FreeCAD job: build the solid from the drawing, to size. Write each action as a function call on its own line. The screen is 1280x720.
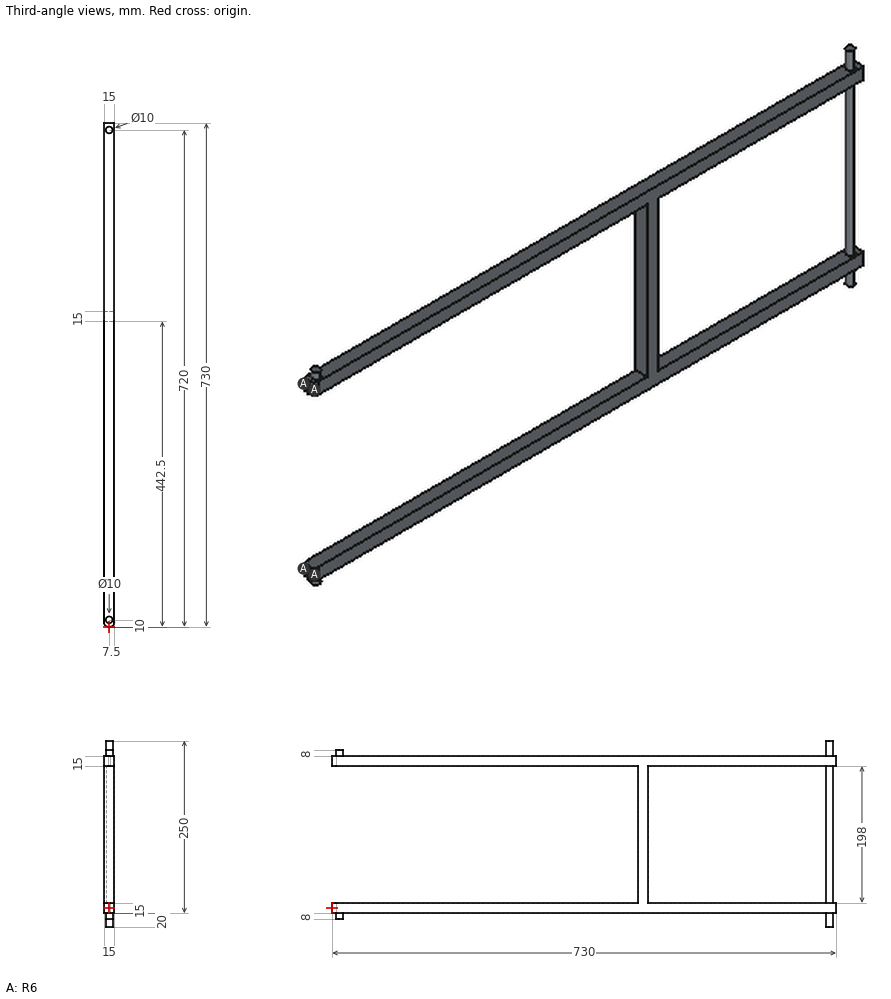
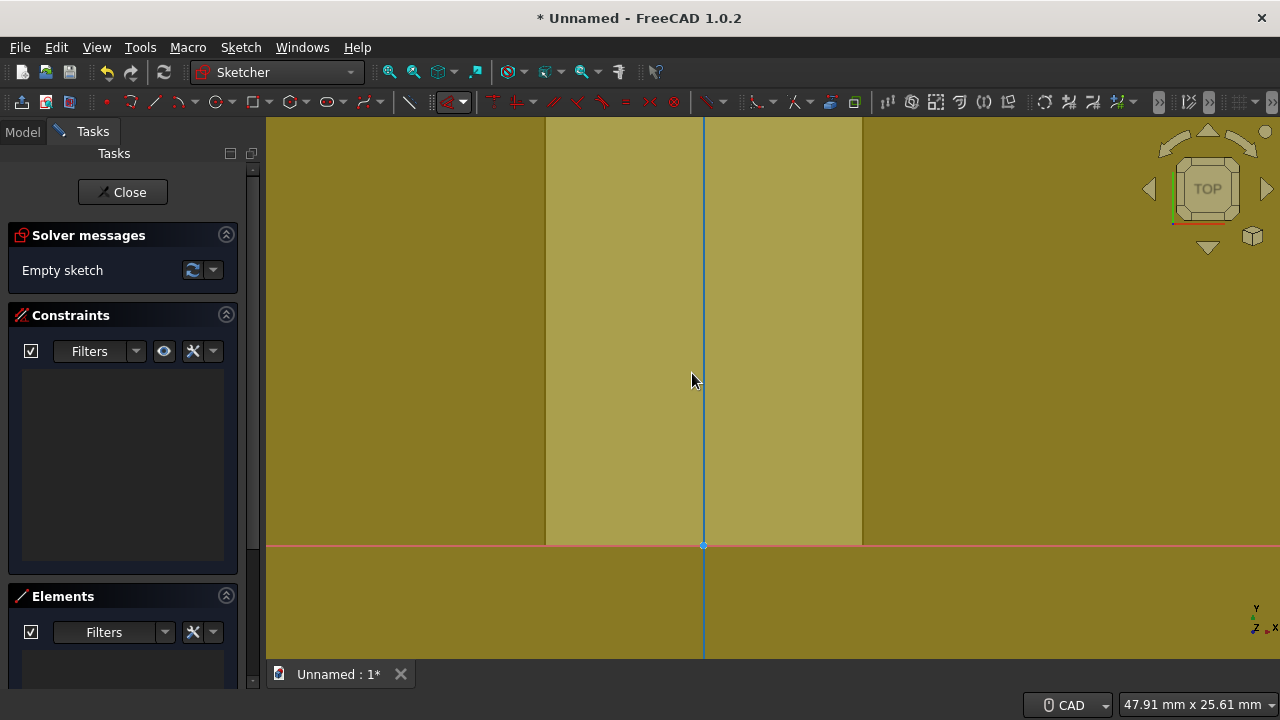
click(216, 102)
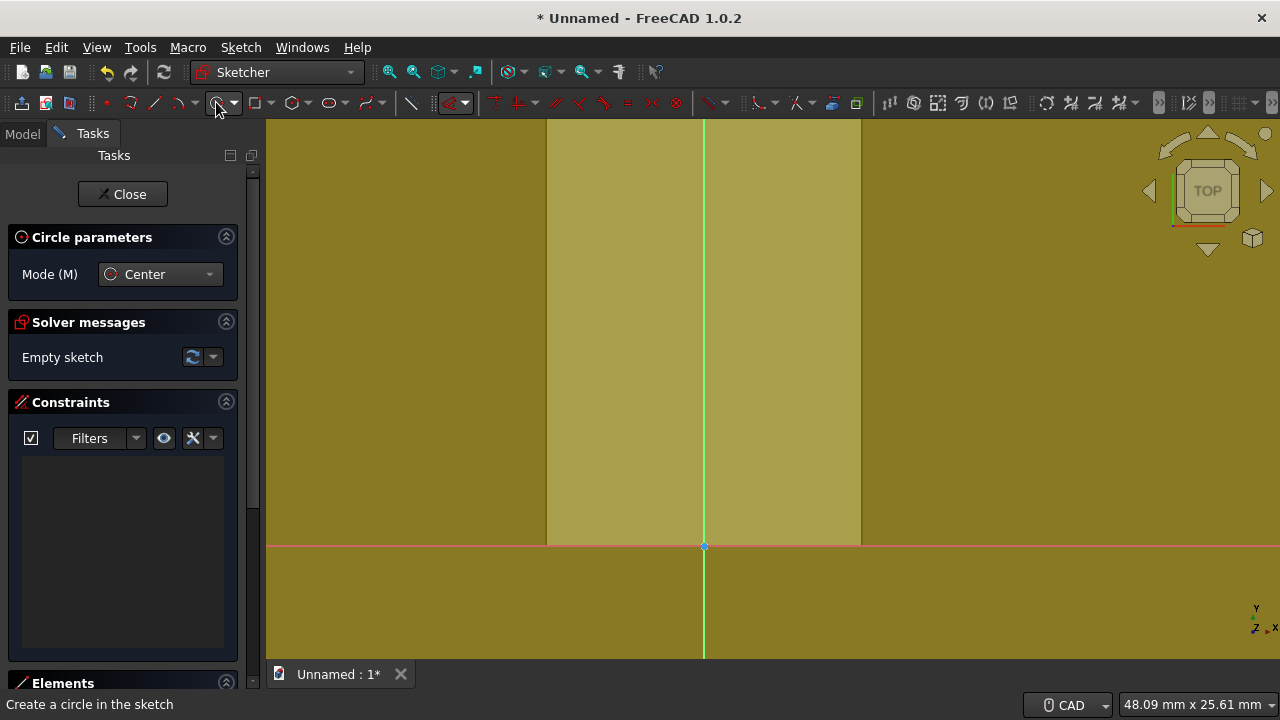
click(704, 335)
move(779, 261)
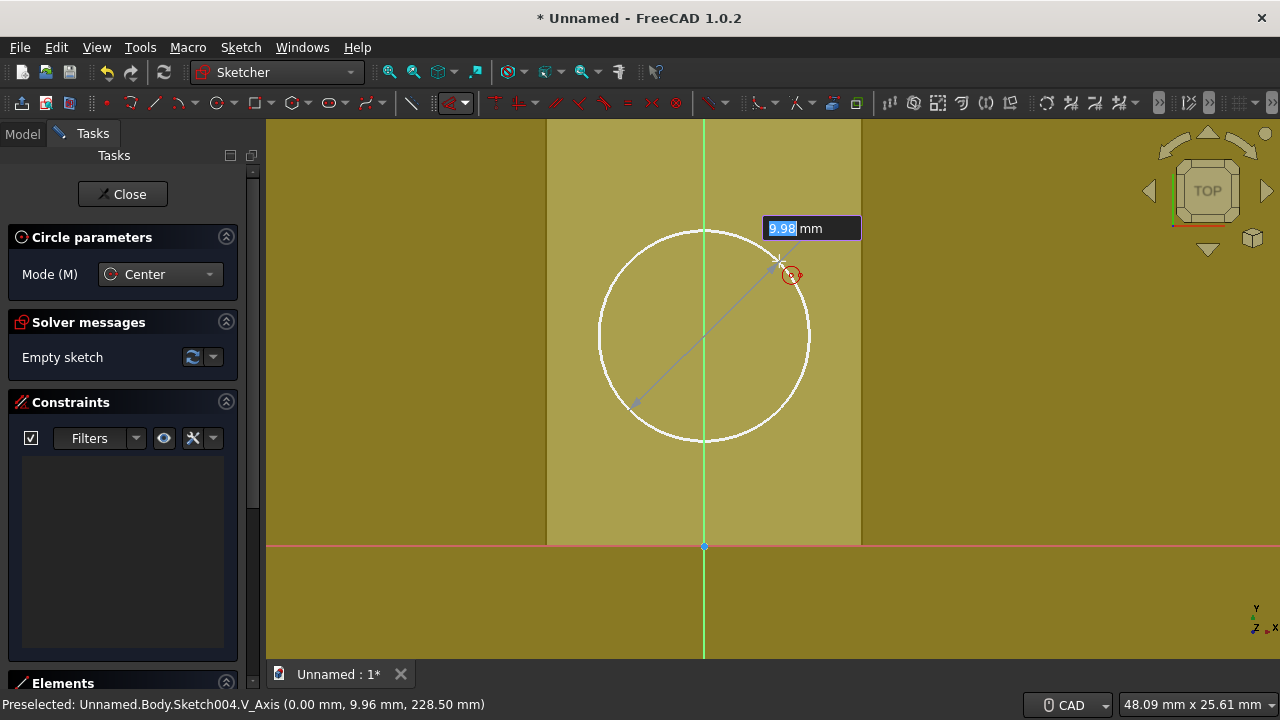
text(10)
key(Return)
key(Escape)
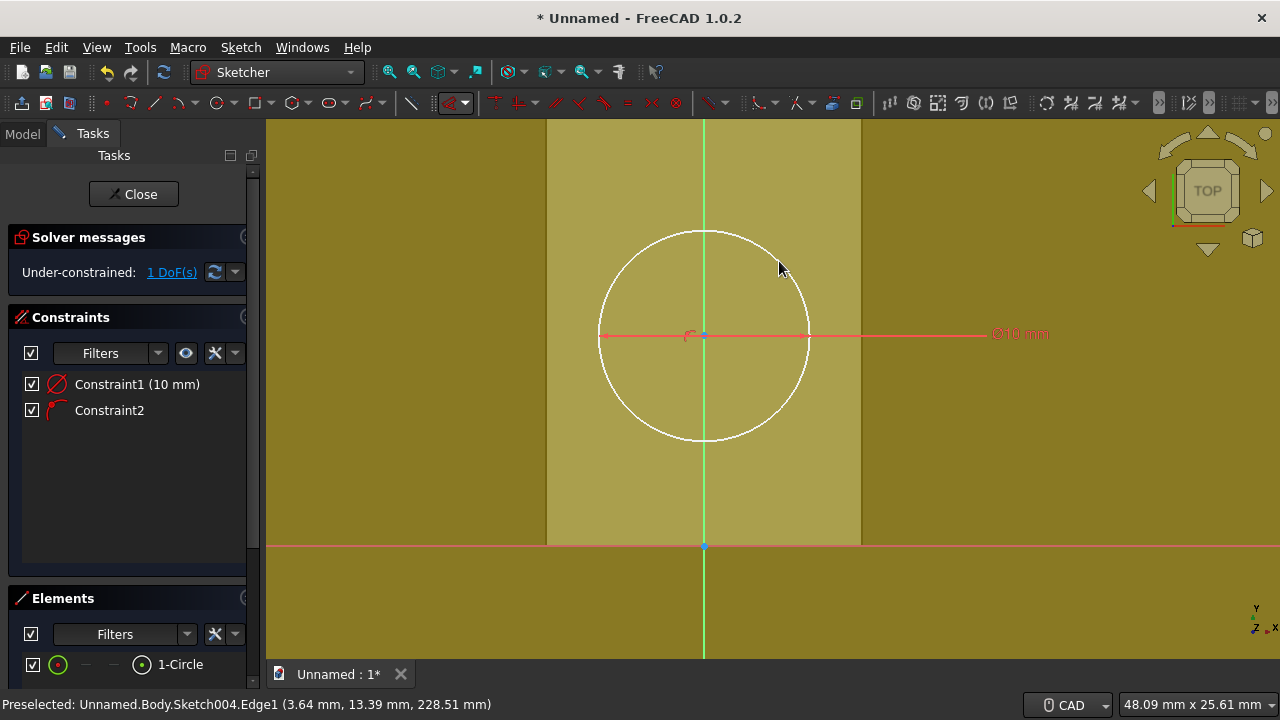
click(704, 336)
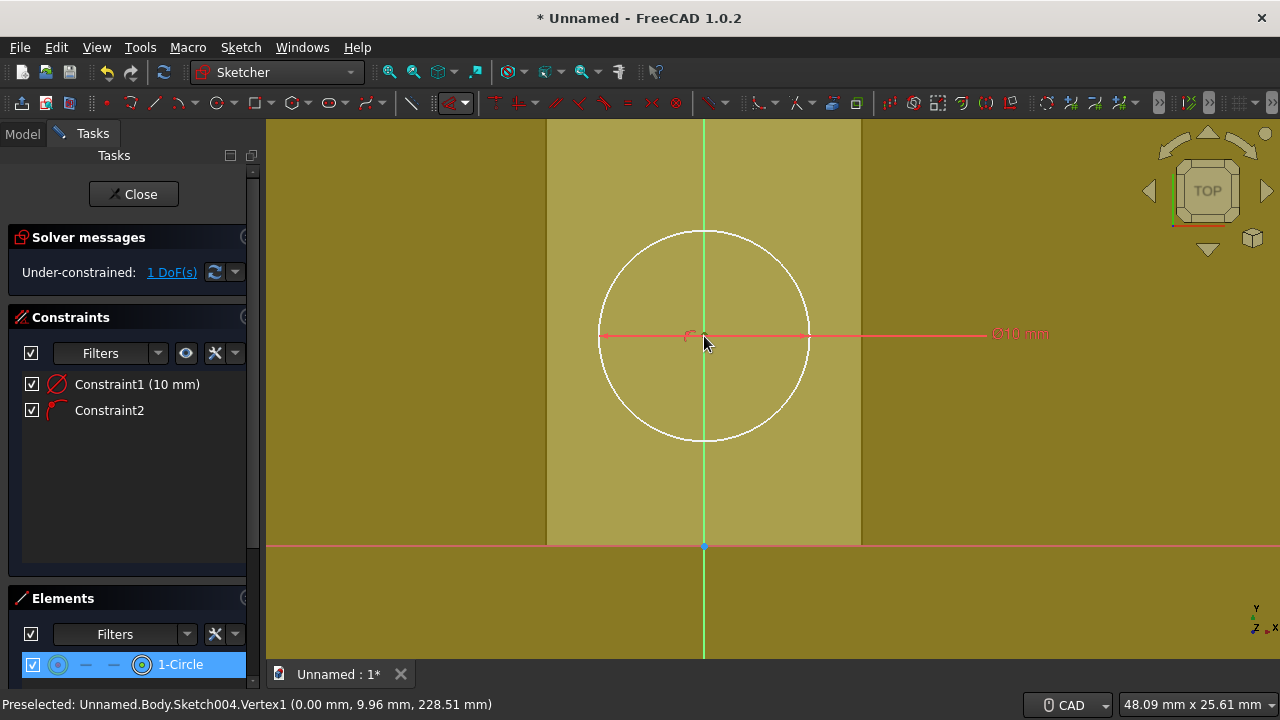
key(i)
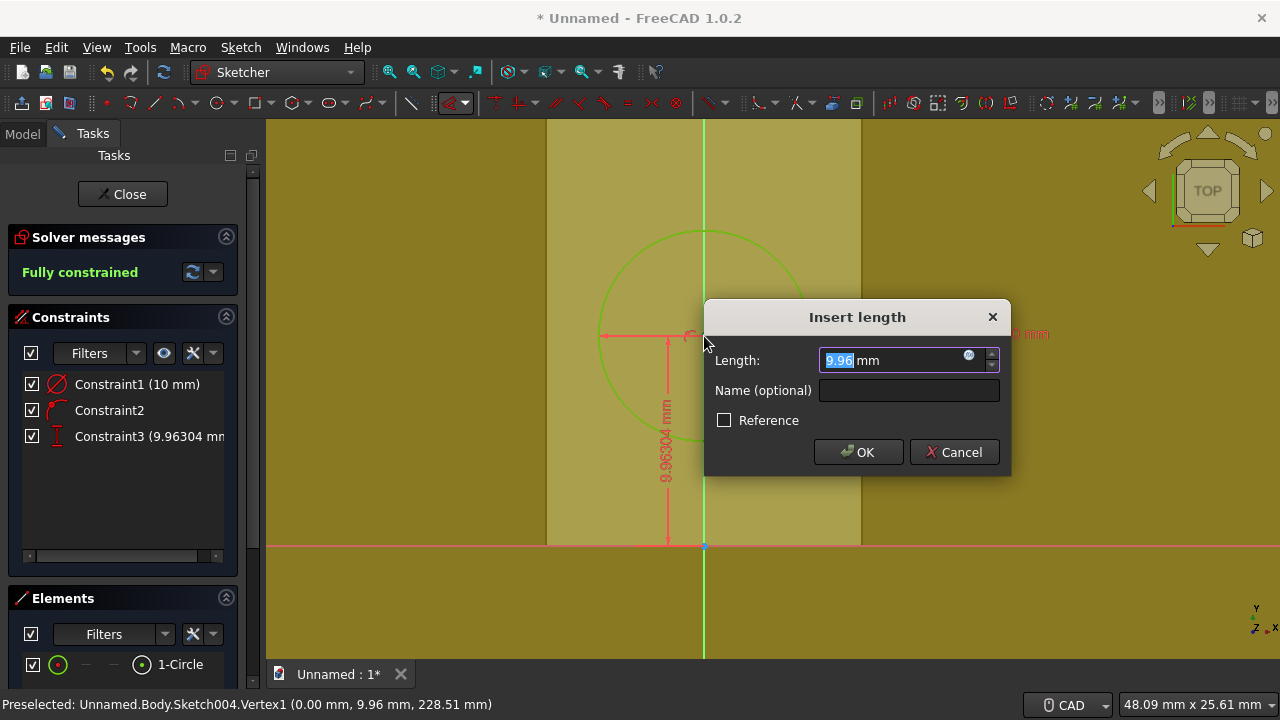
text(10)
key(Return)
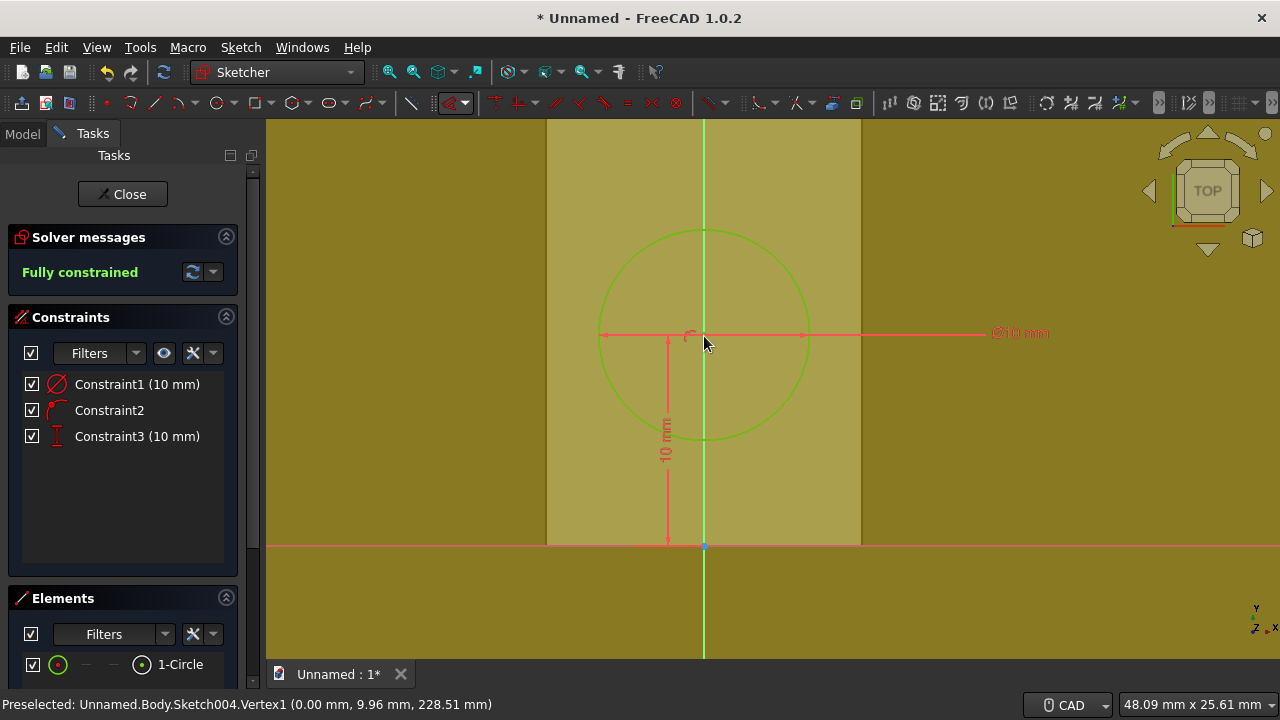
click(123, 194)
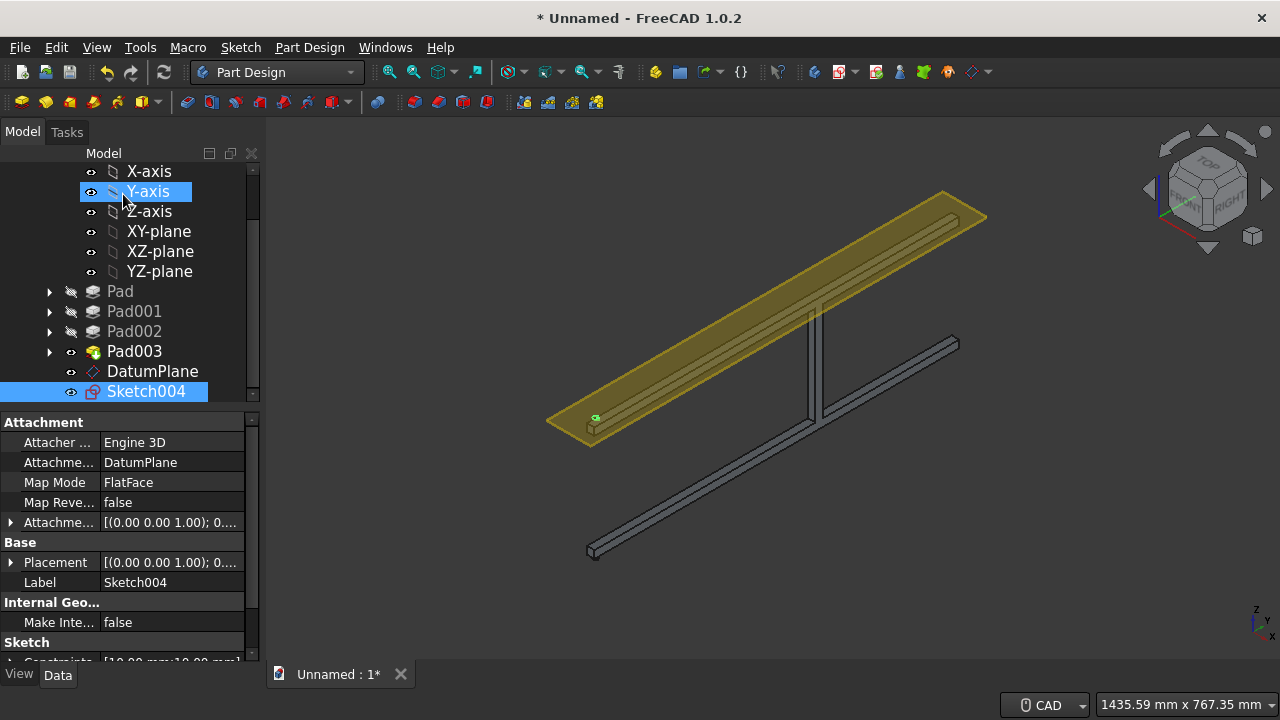
click(22, 102)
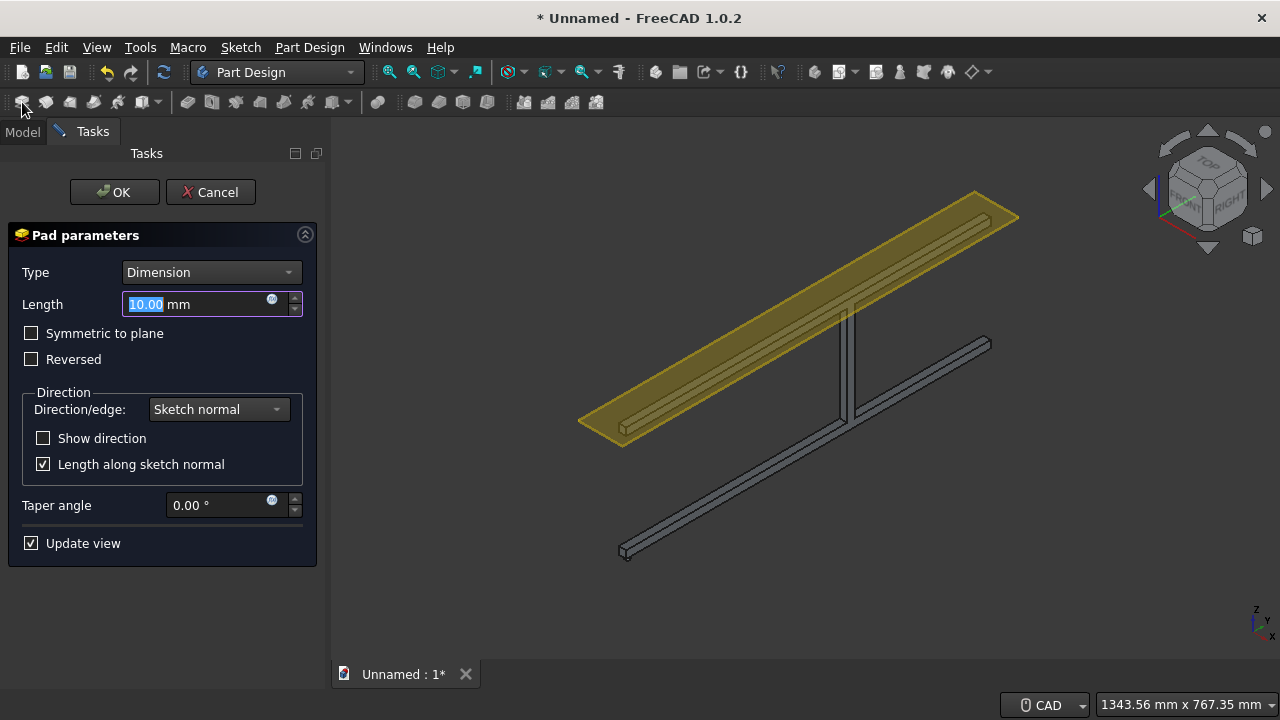
text(8)
key(Tab)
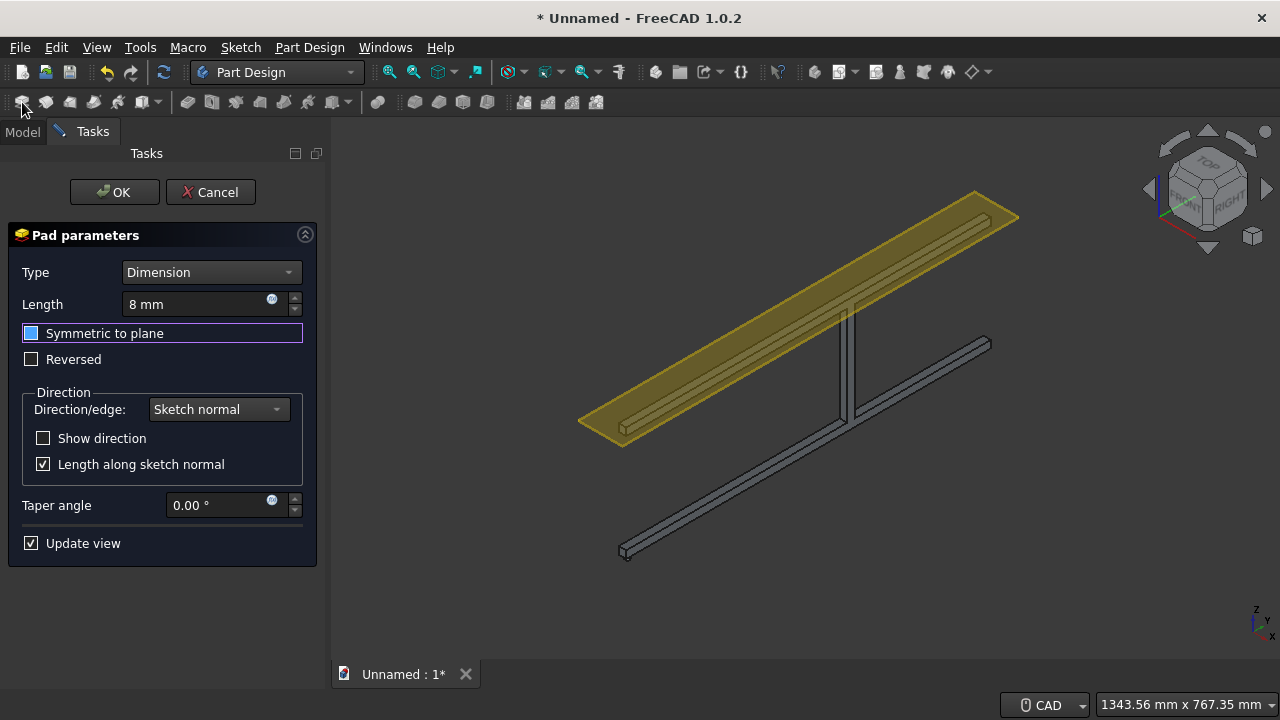
click(30, 359)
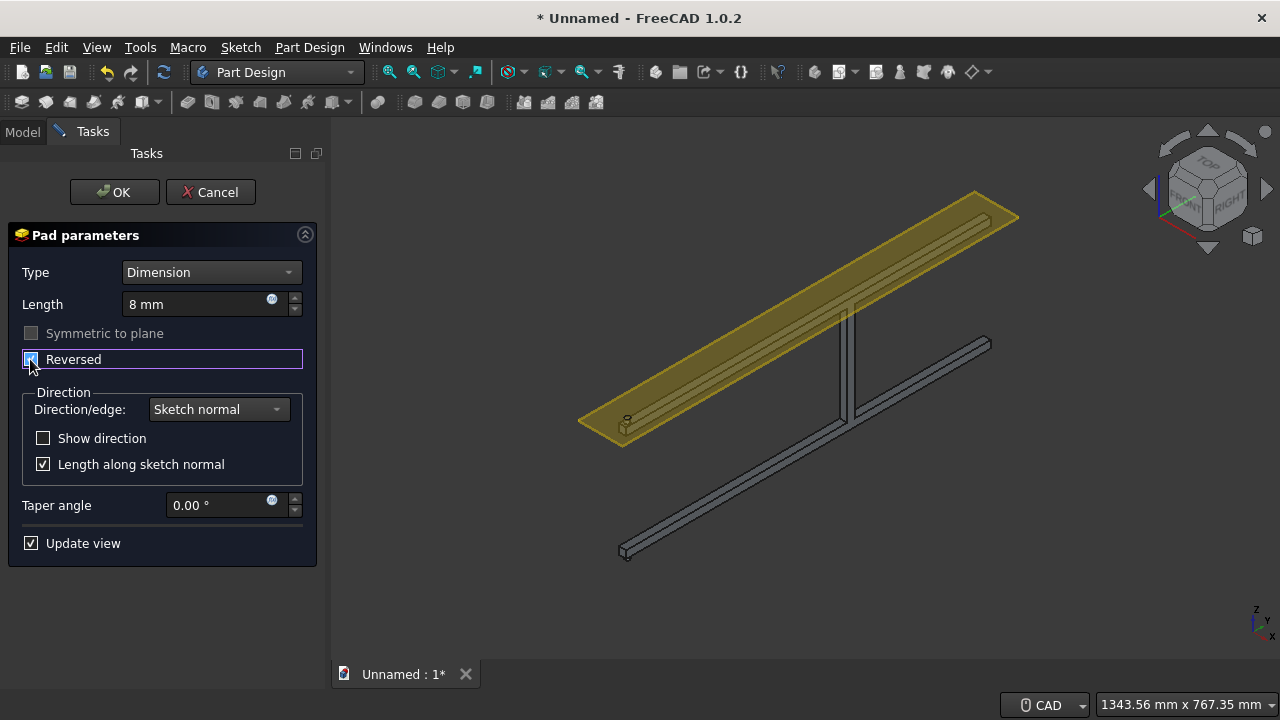
click(115, 192)